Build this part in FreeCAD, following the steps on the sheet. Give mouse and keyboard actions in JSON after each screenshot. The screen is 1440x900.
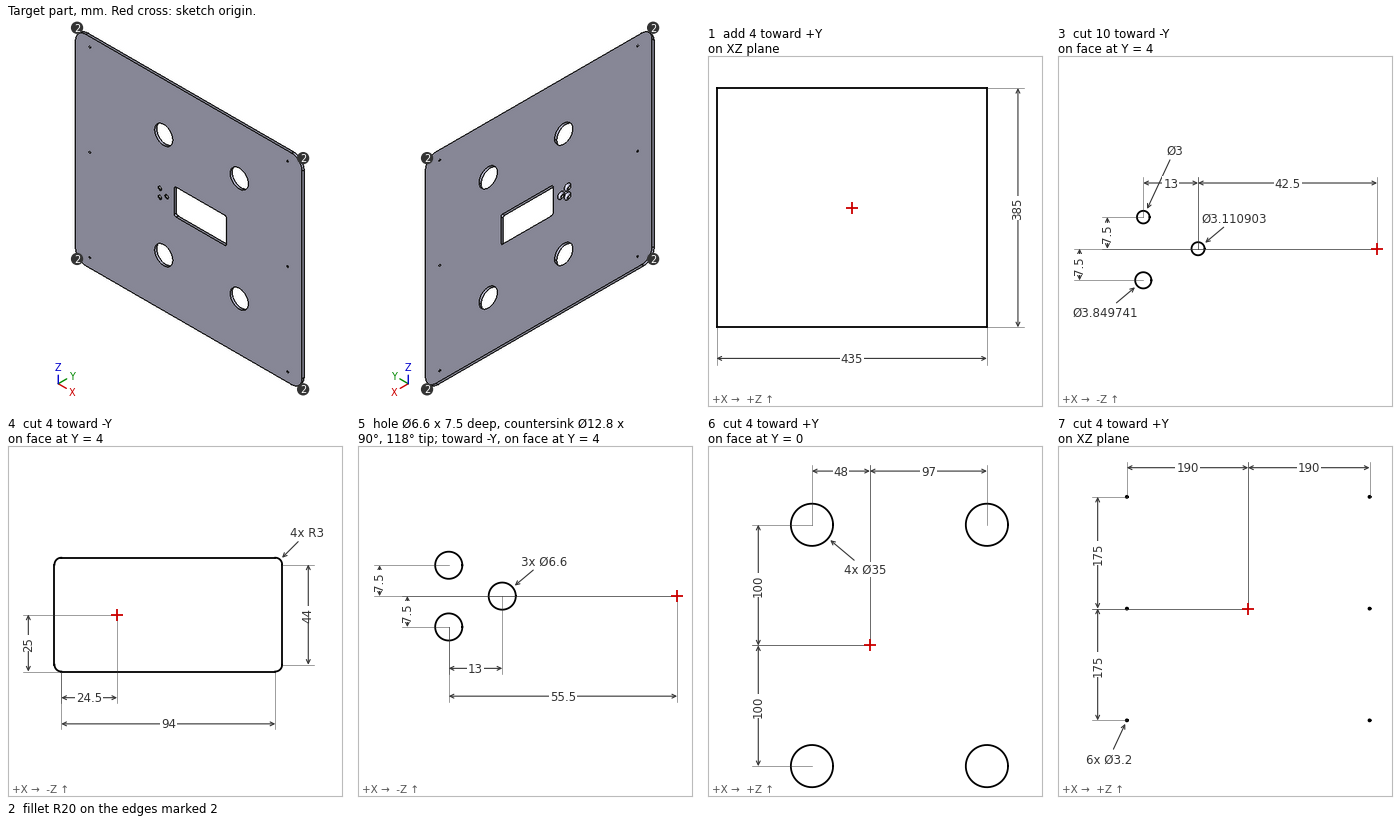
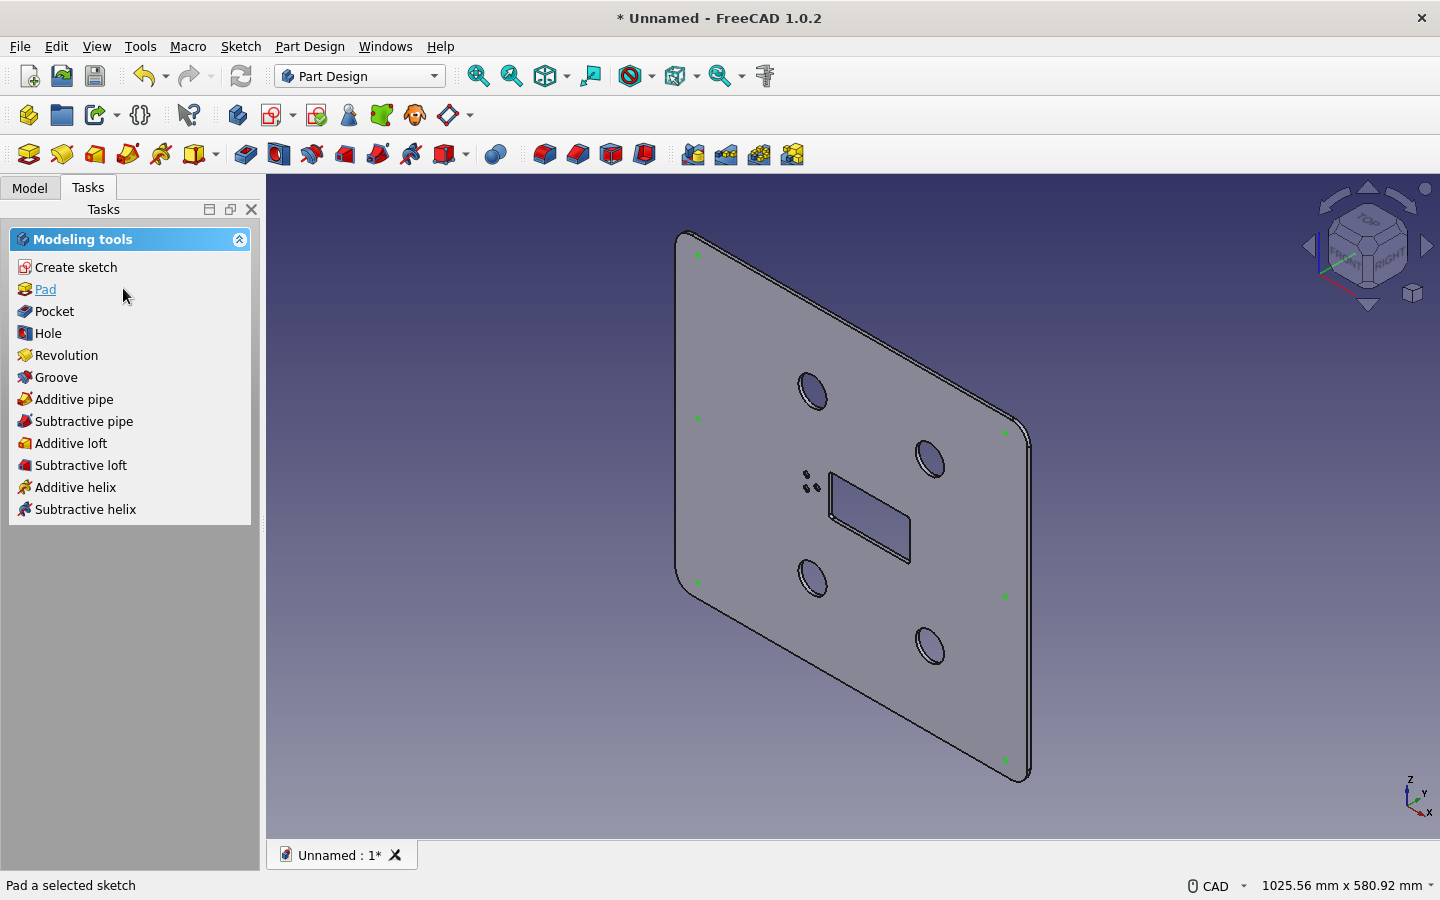
{"action": "left_click", "coordinate": [246, 154]}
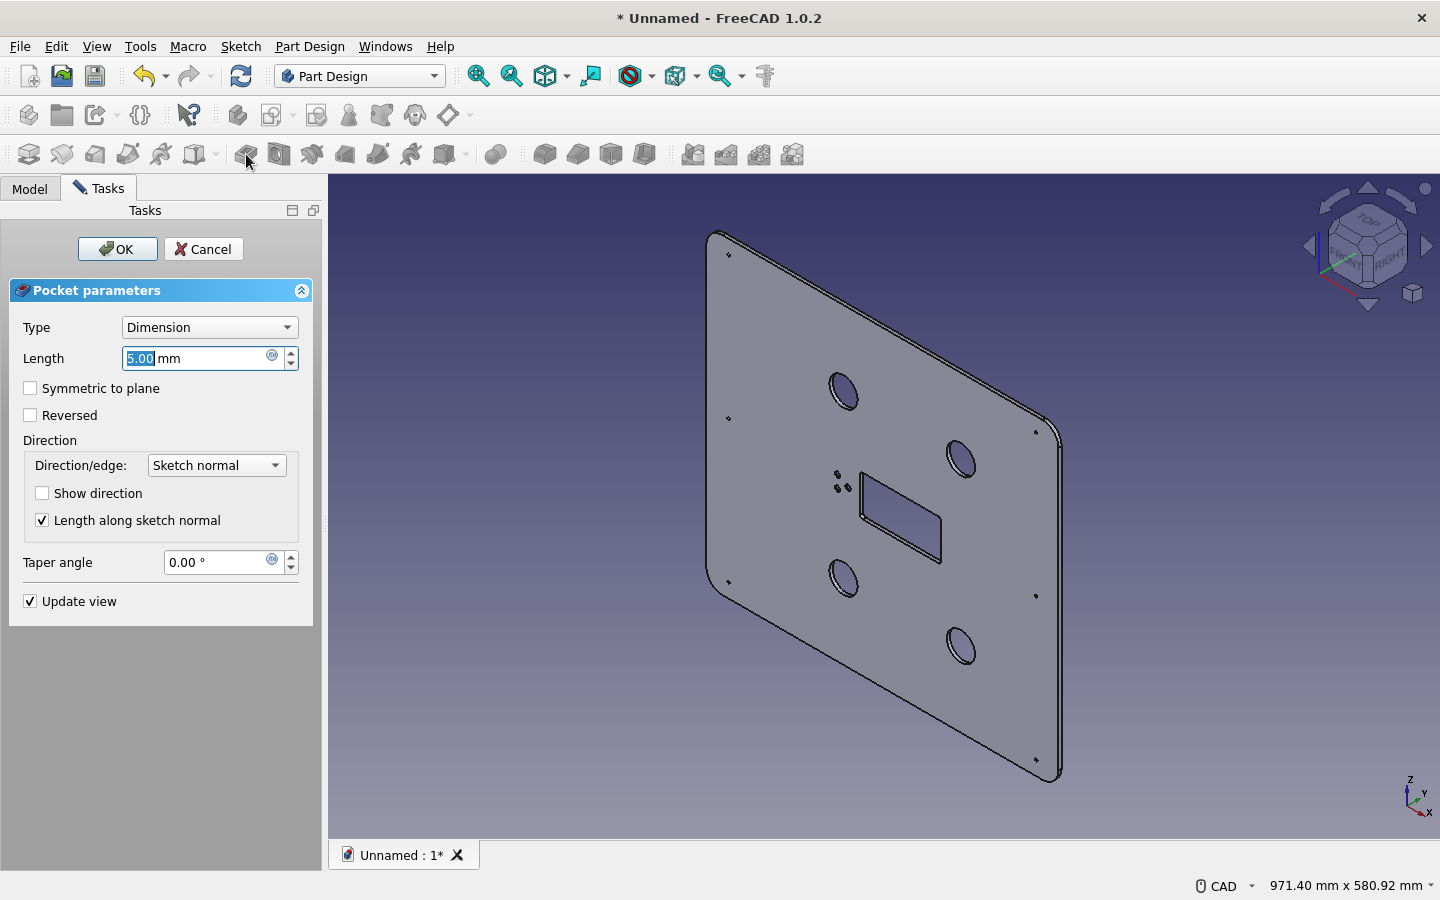
{"action": "type", "text": "4"}
{"action": "key", "text": "Tab"}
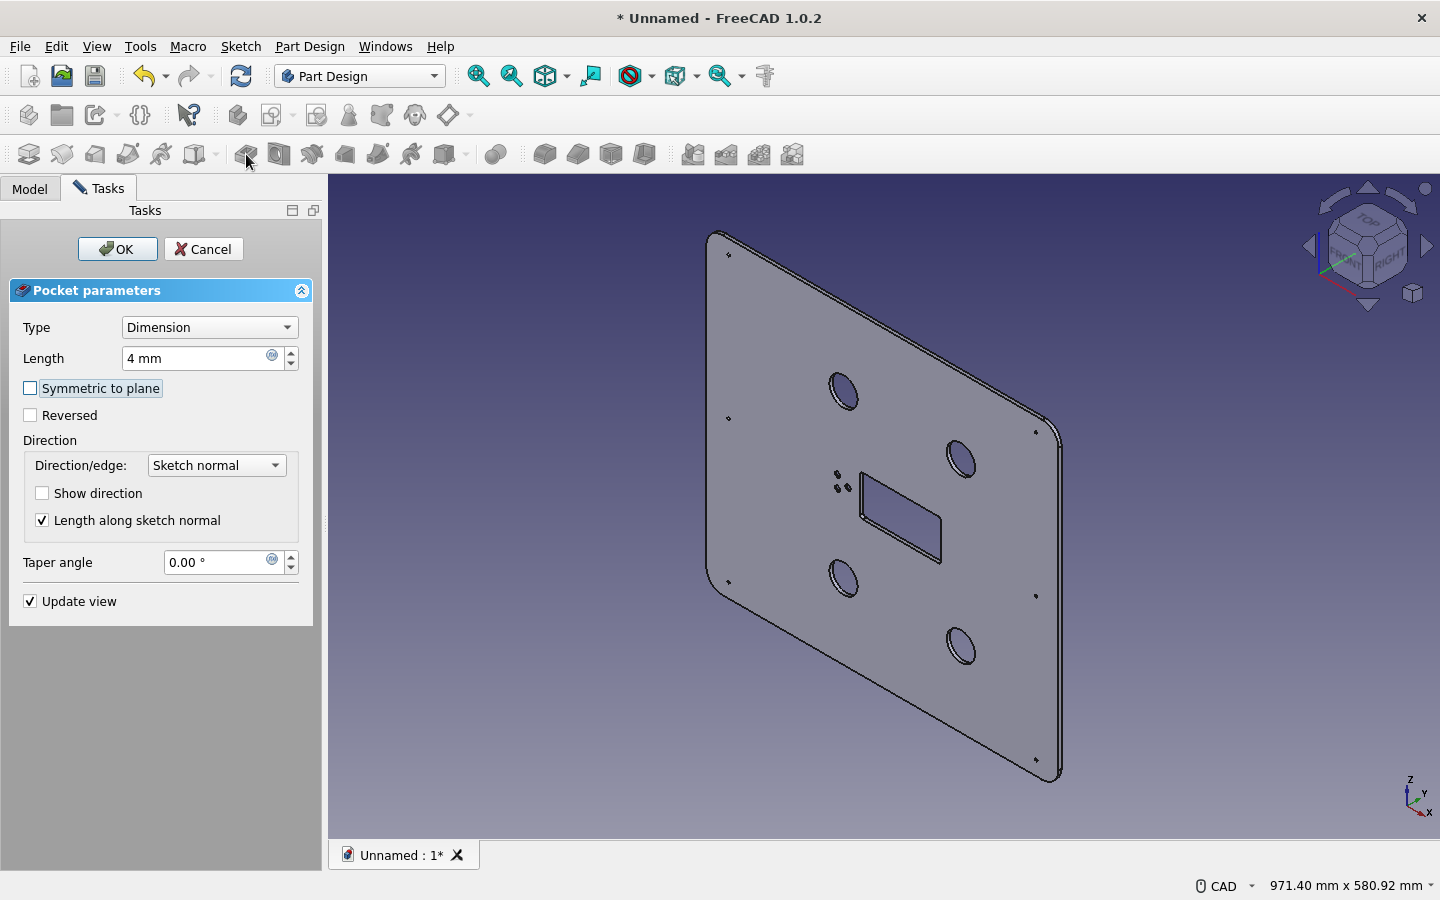
{"action": "left_click", "coordinate": [118, 249]}